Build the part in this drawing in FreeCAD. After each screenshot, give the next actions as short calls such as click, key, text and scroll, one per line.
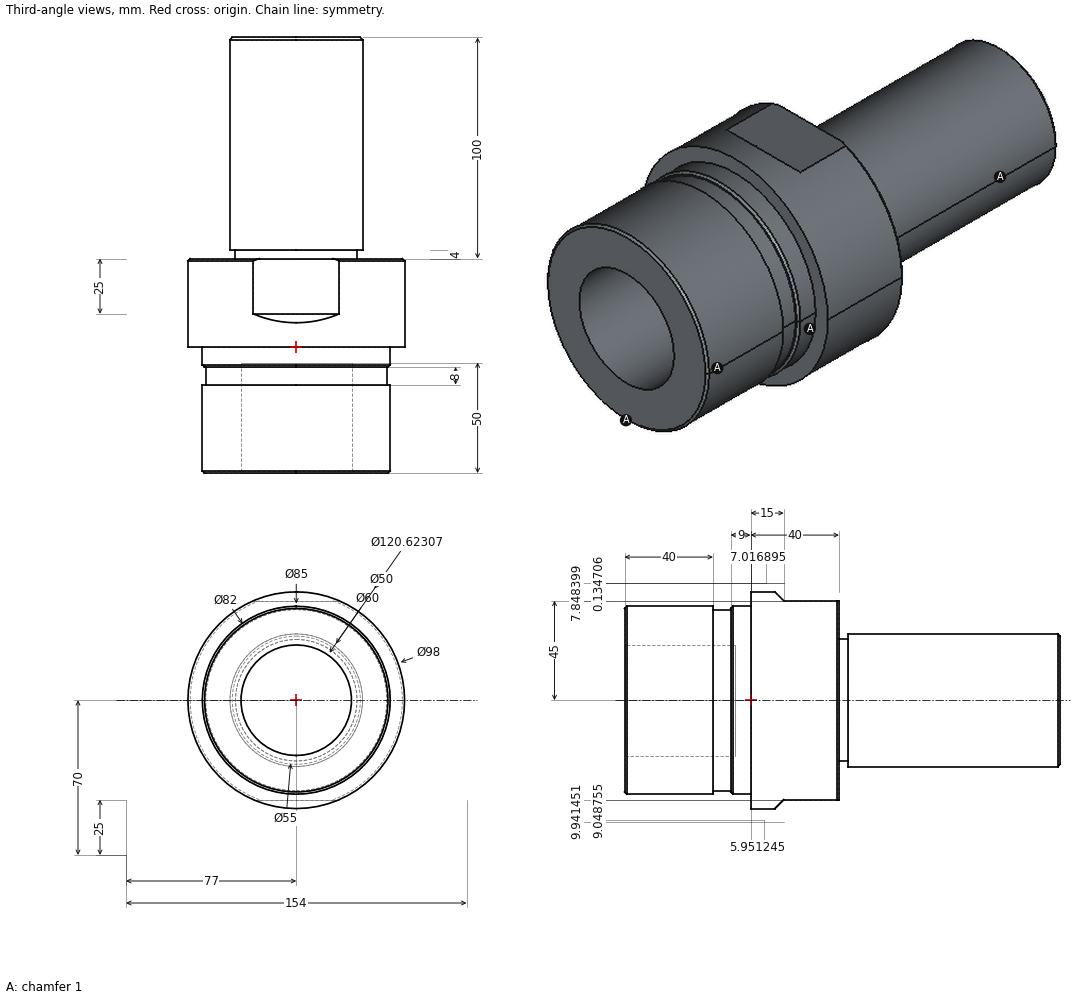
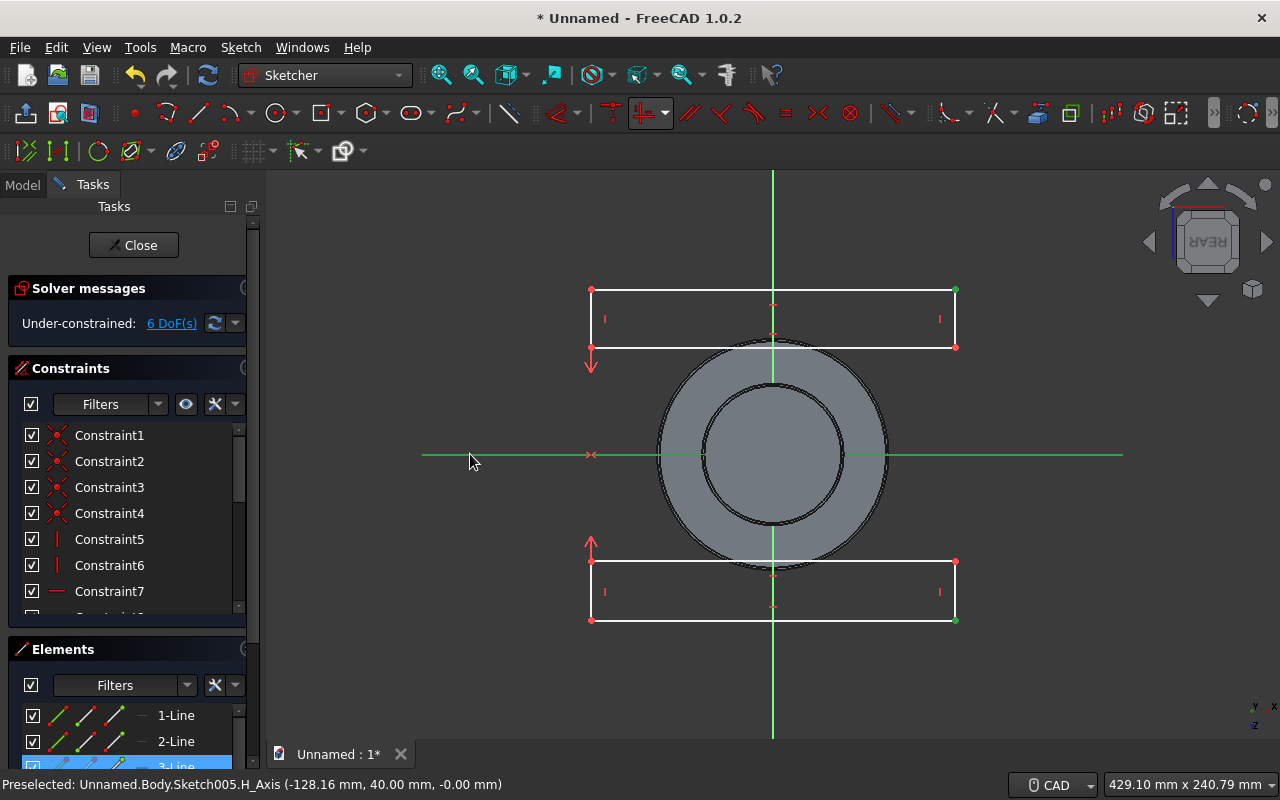
click(818, 114)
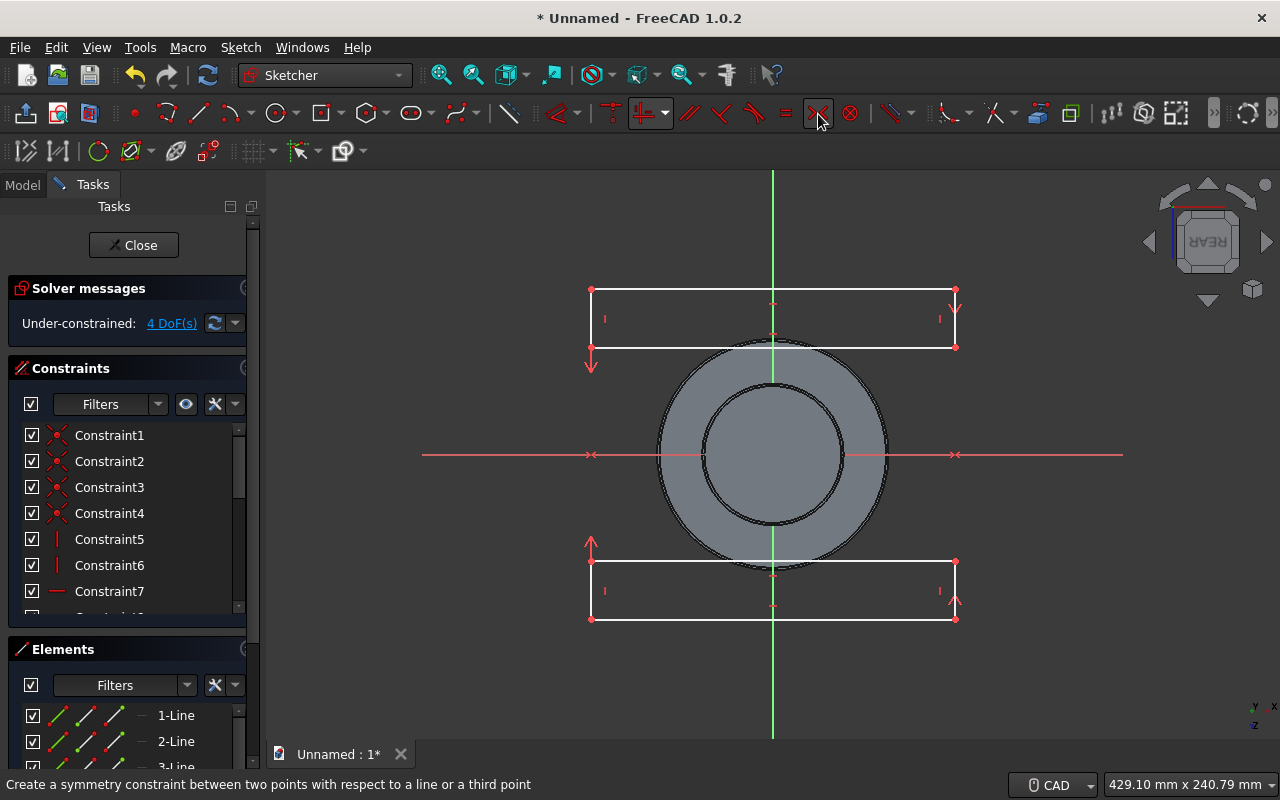
click(556, 114)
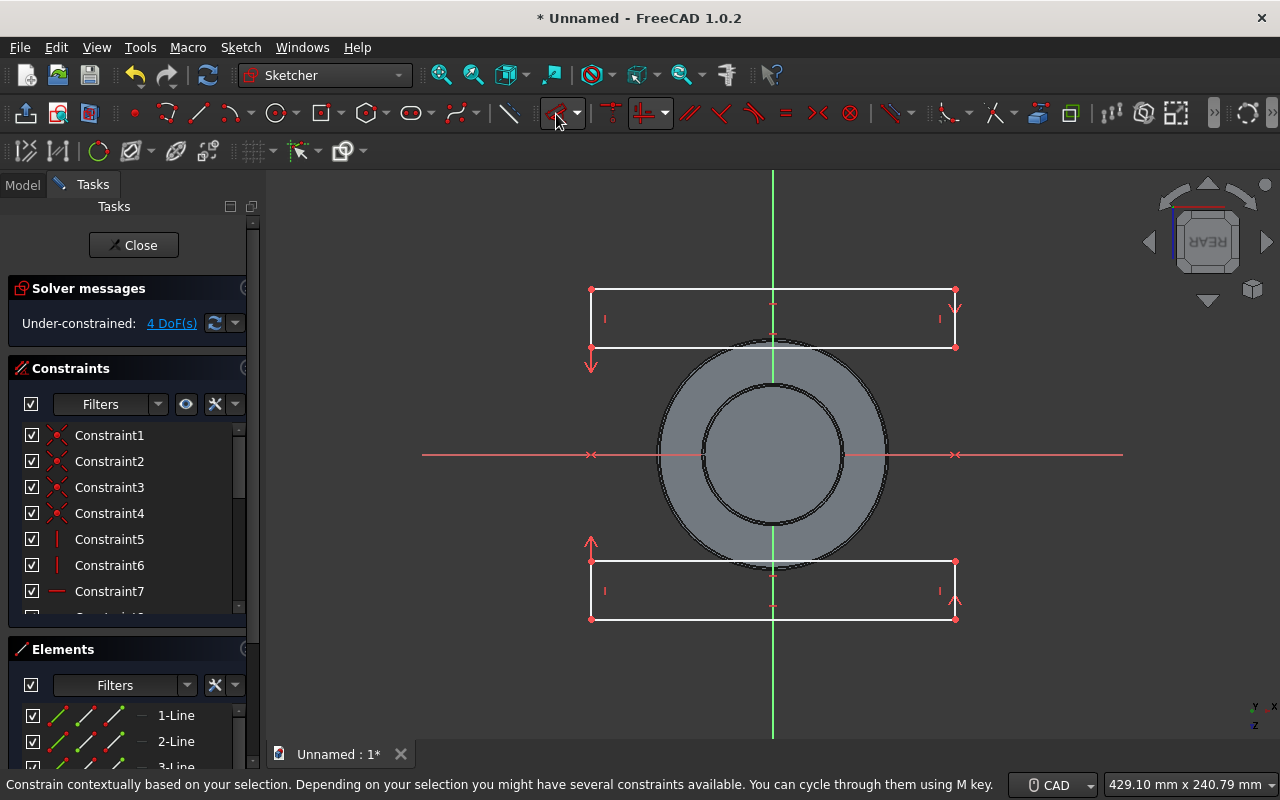
click(591, 307)
click(557, 318)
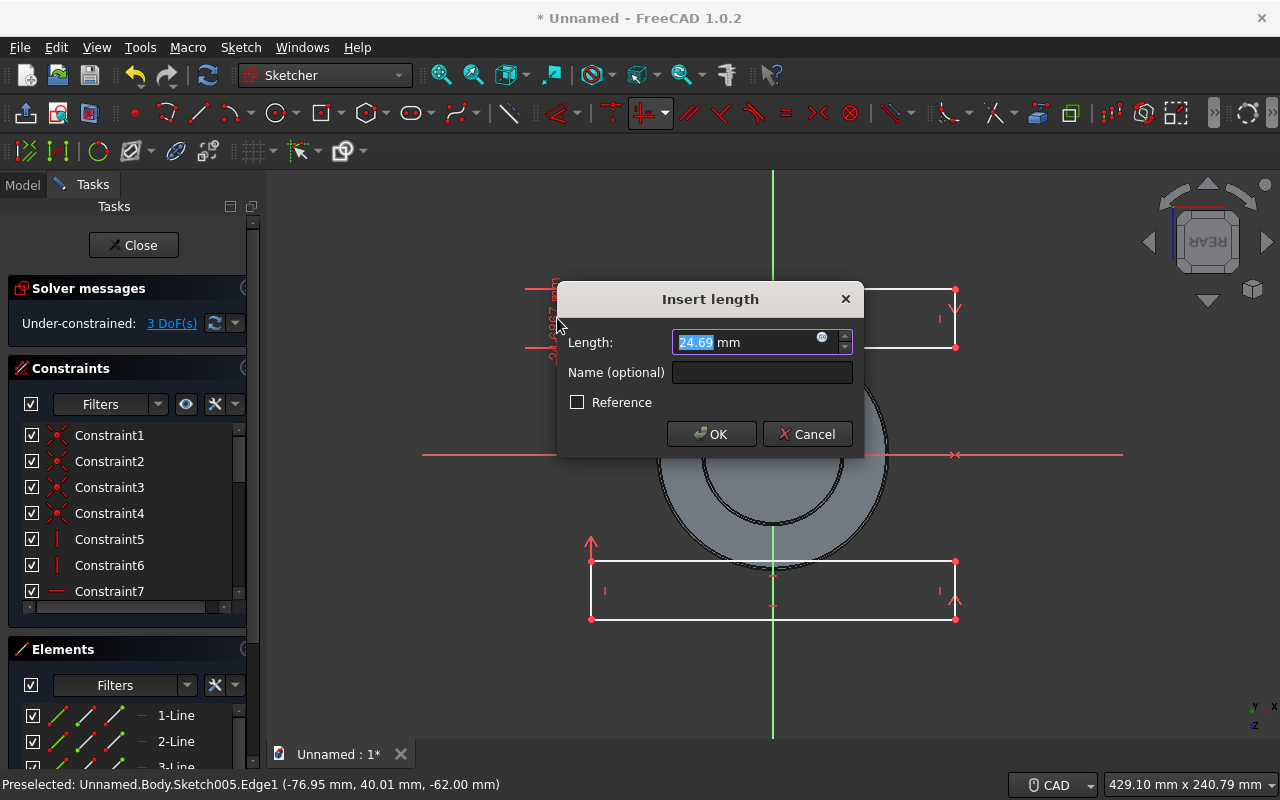
text(25)
key(Return)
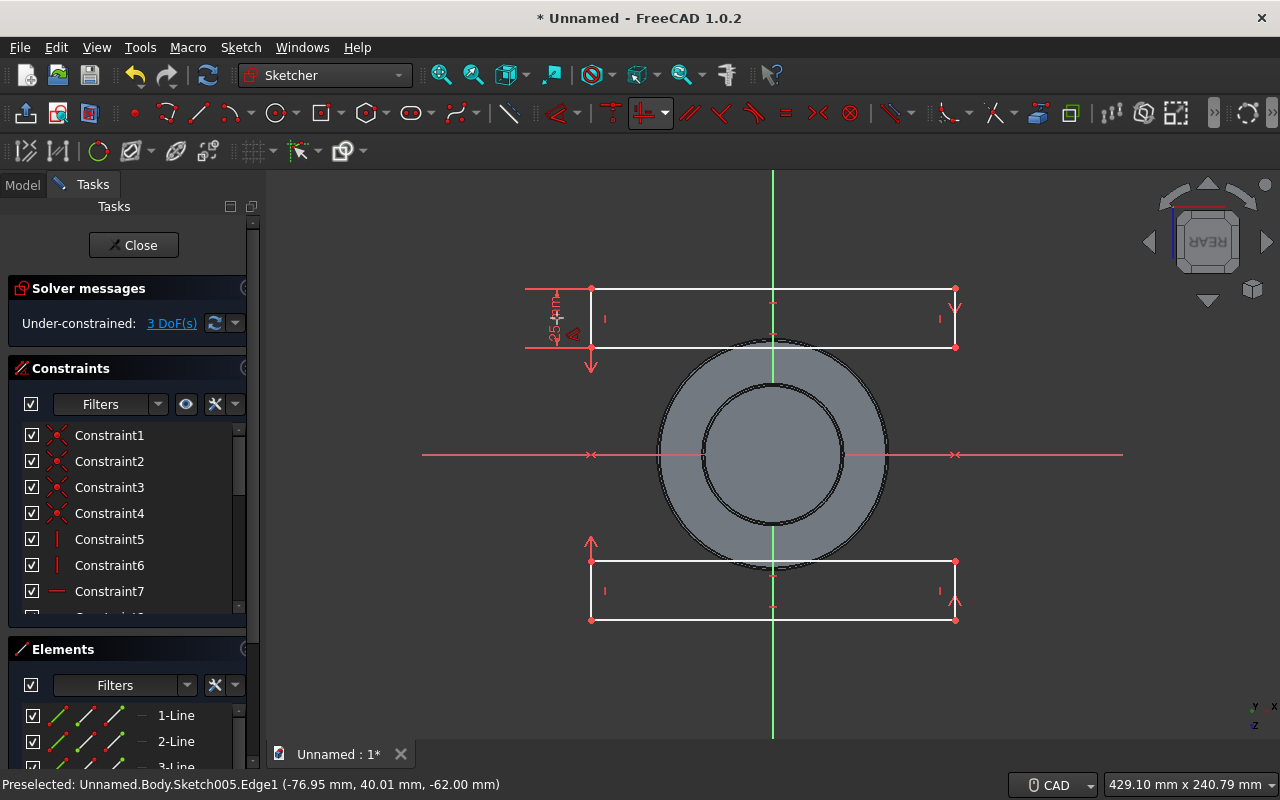
click(700, 348)
click(689, 314)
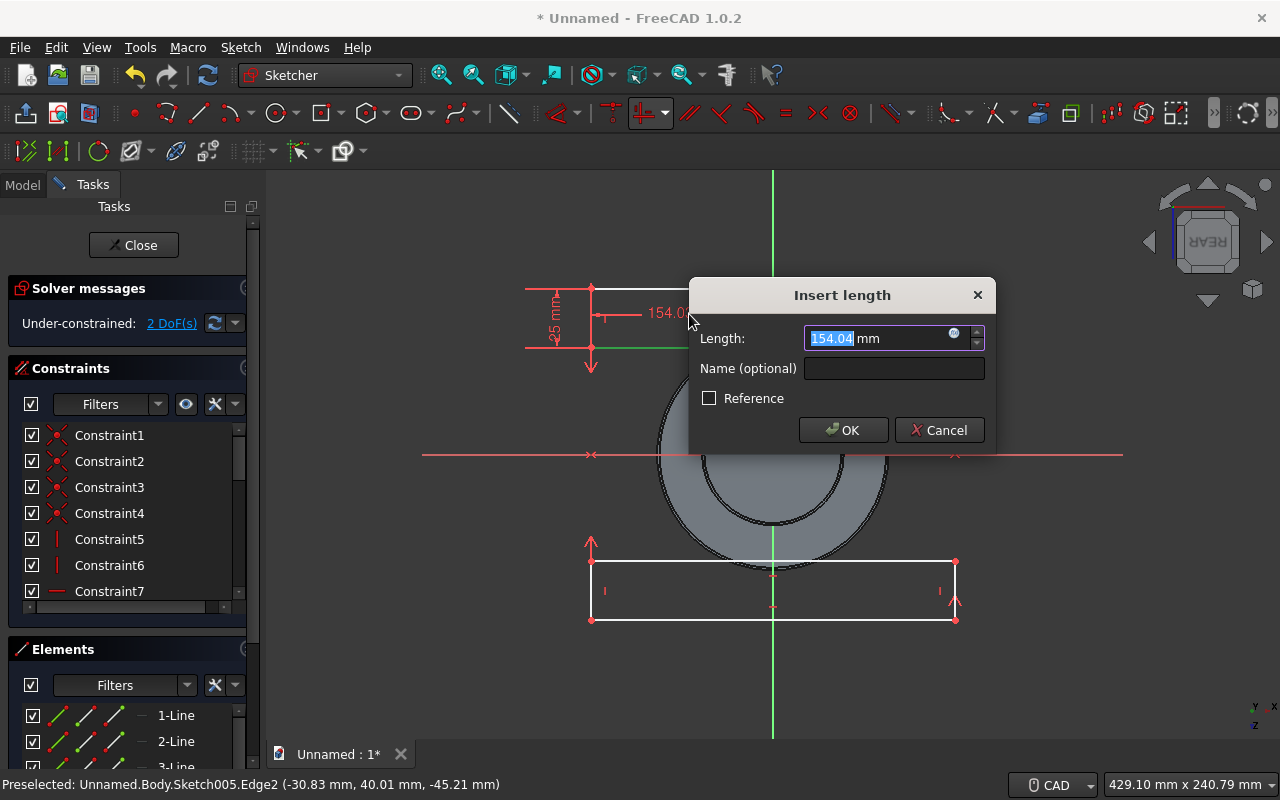
text(154)
key(Return)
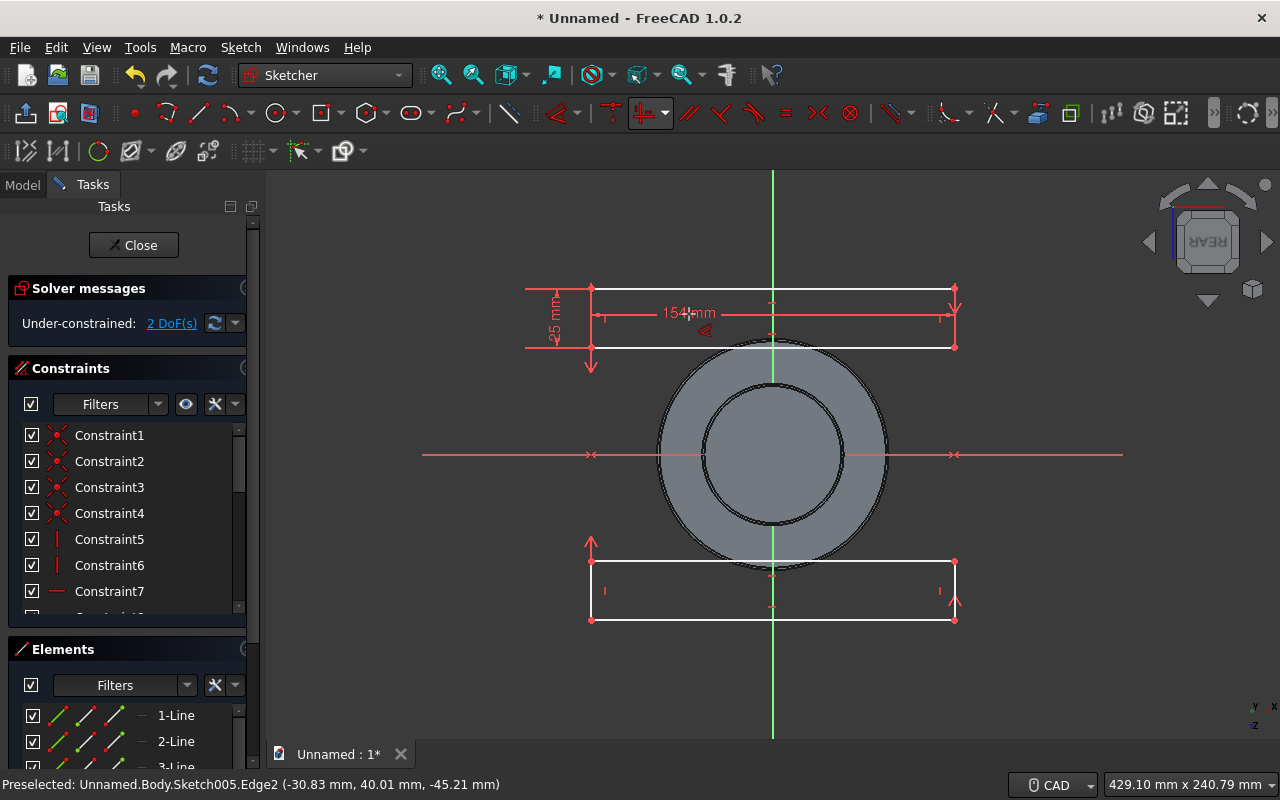
click(591, 289)
click(682, 255)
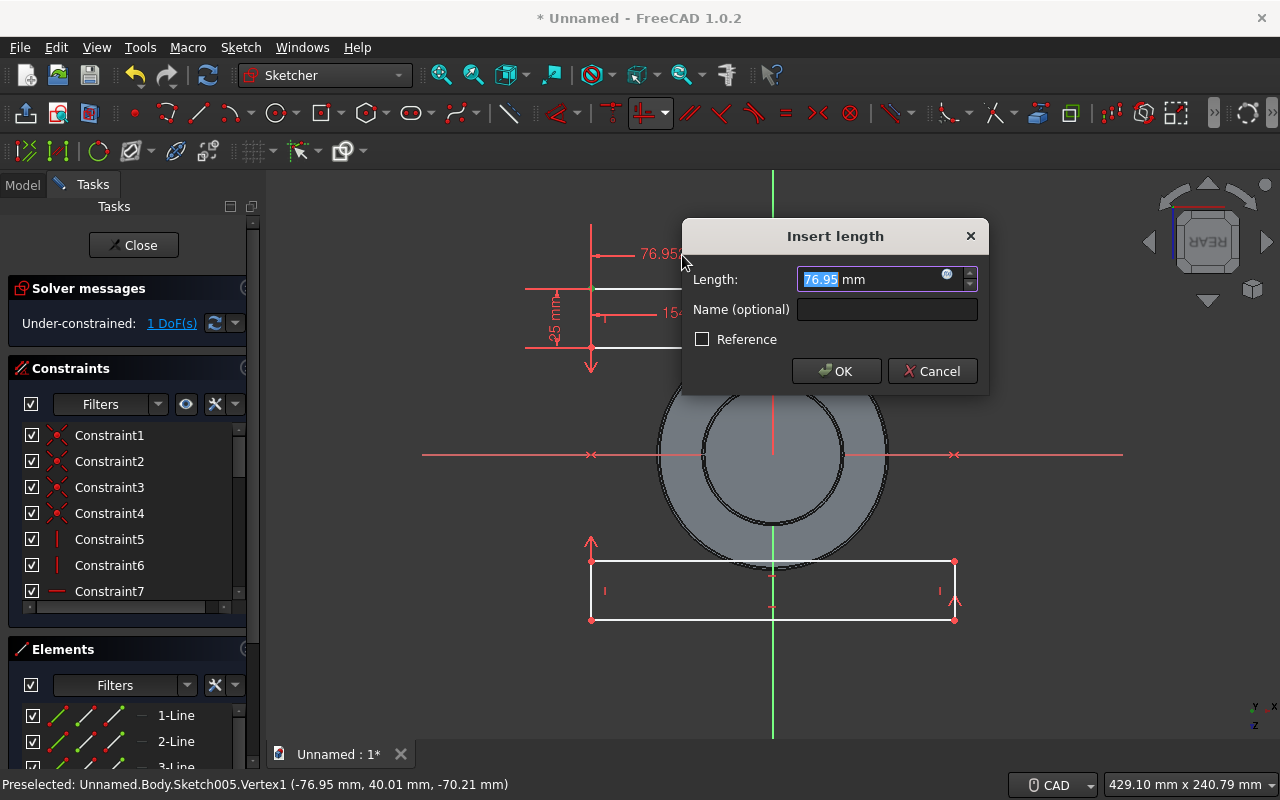
text(77)
key(Return)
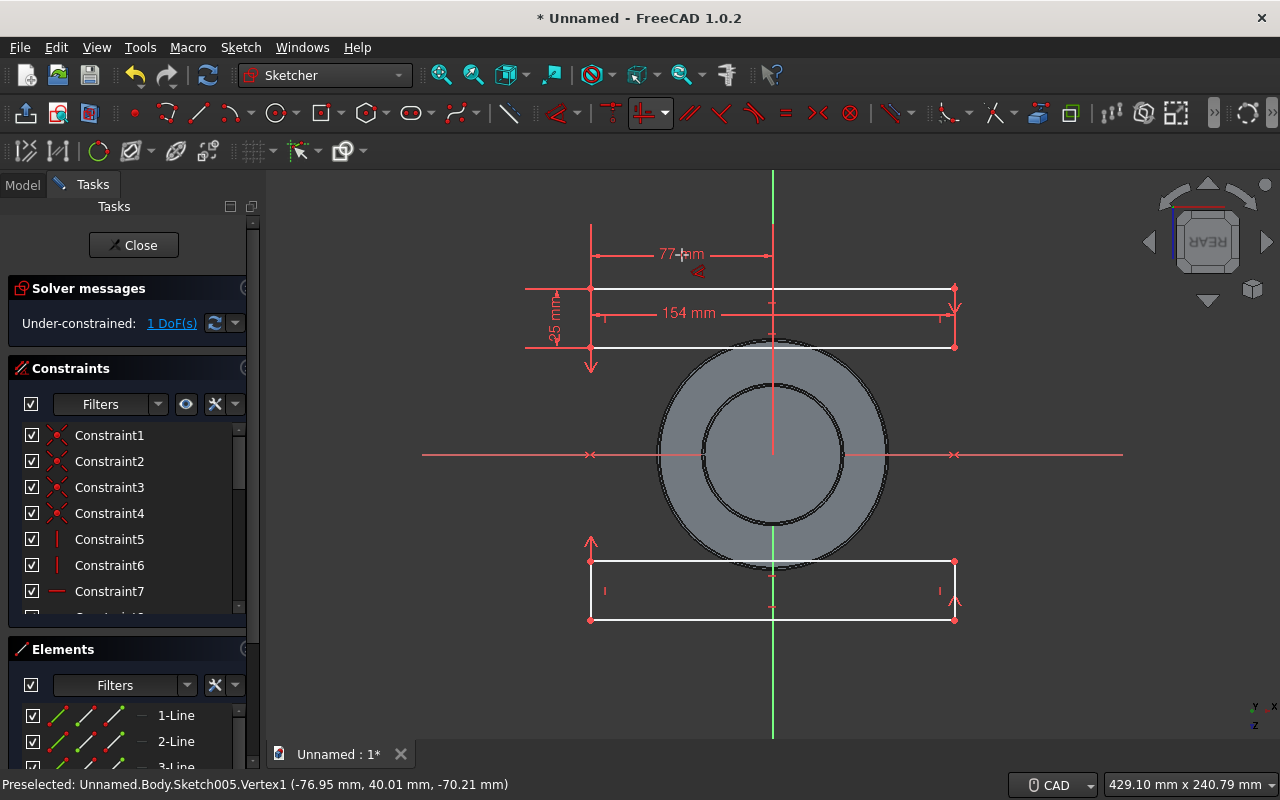
click(591, 289)
click(557, 372)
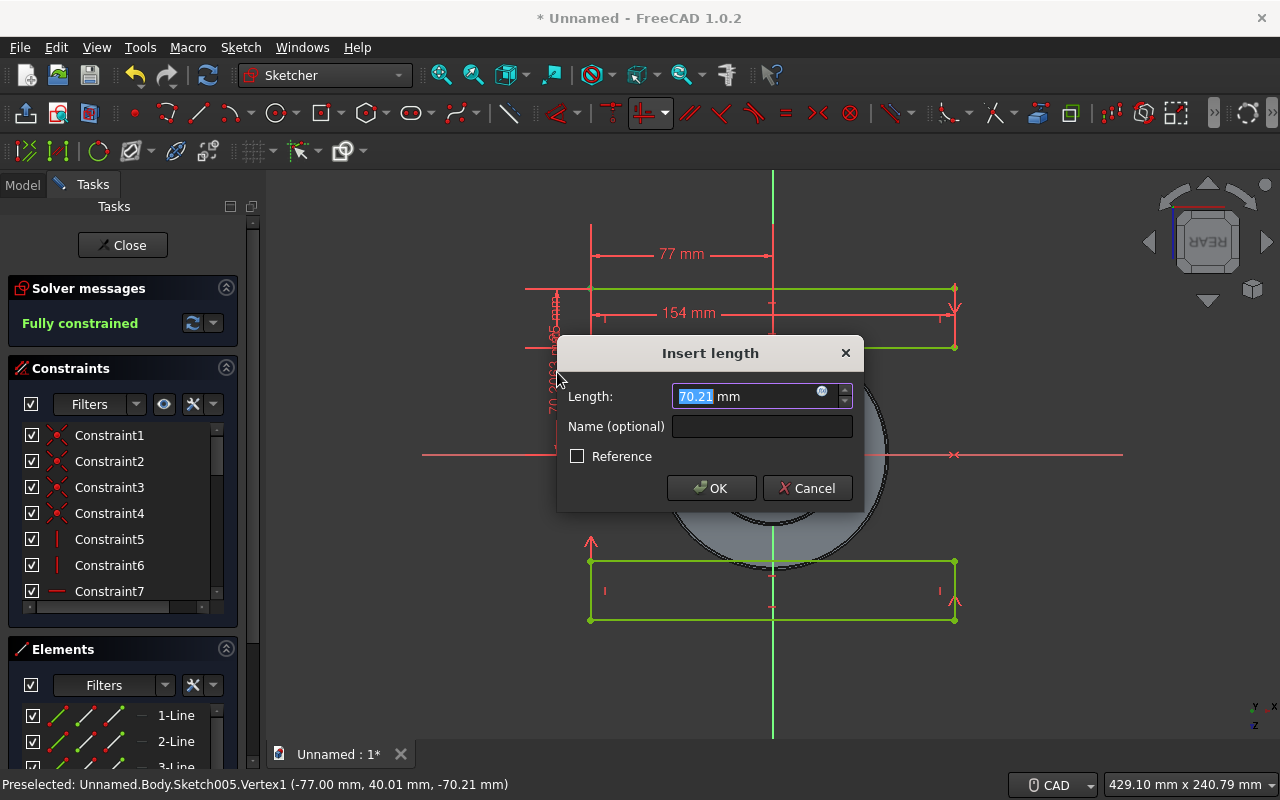
text(70)
key(Return)
key(Escape)